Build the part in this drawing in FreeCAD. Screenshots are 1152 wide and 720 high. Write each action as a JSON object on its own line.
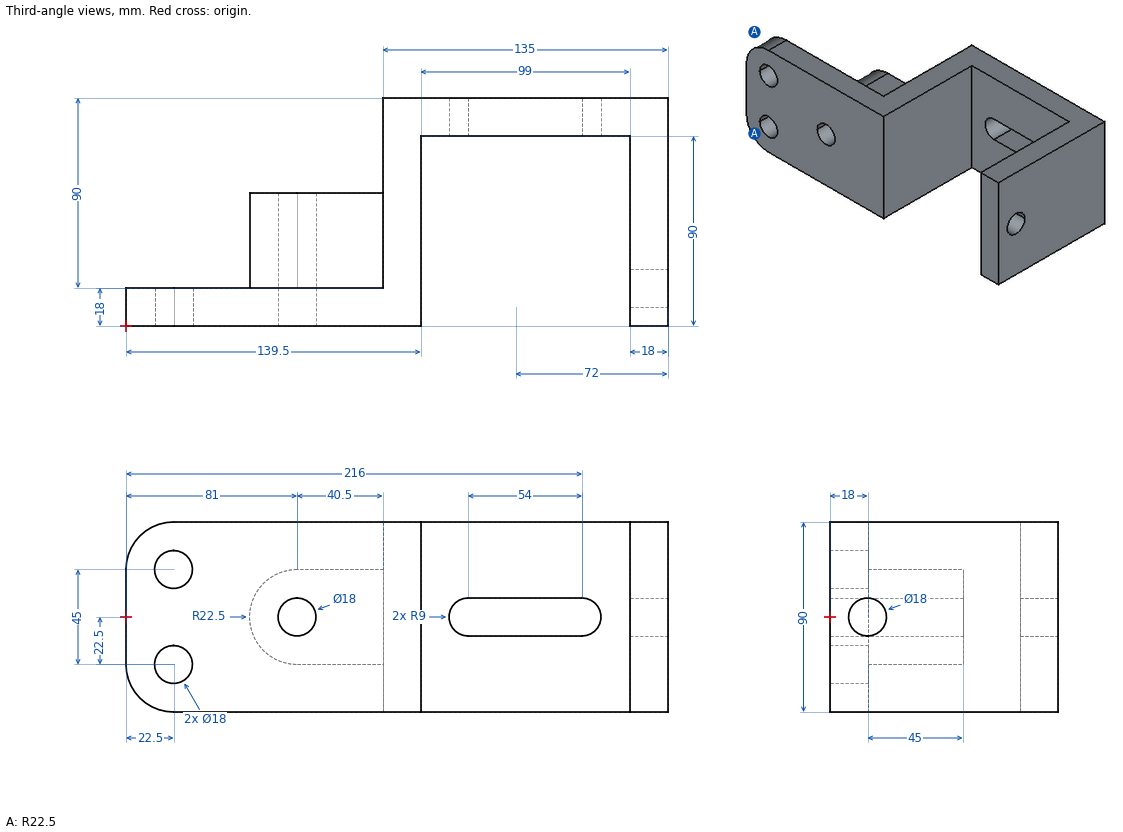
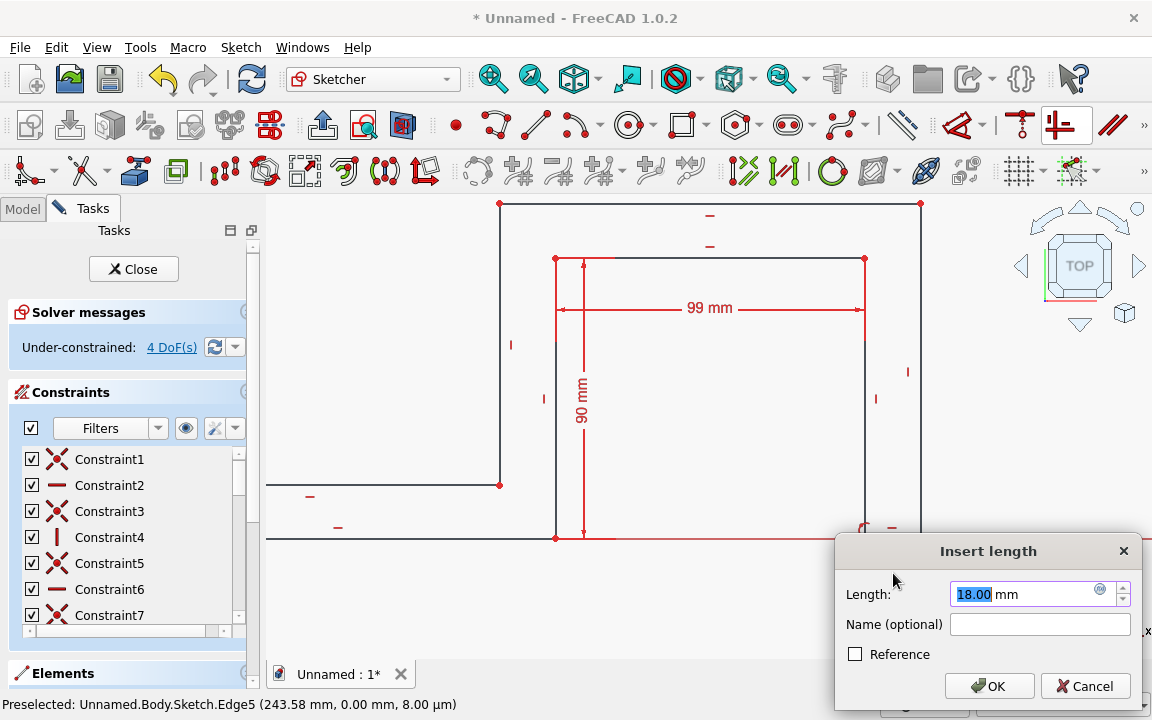
{"action": "type", "text": "18"}
{"action": "key", "text": "Return"}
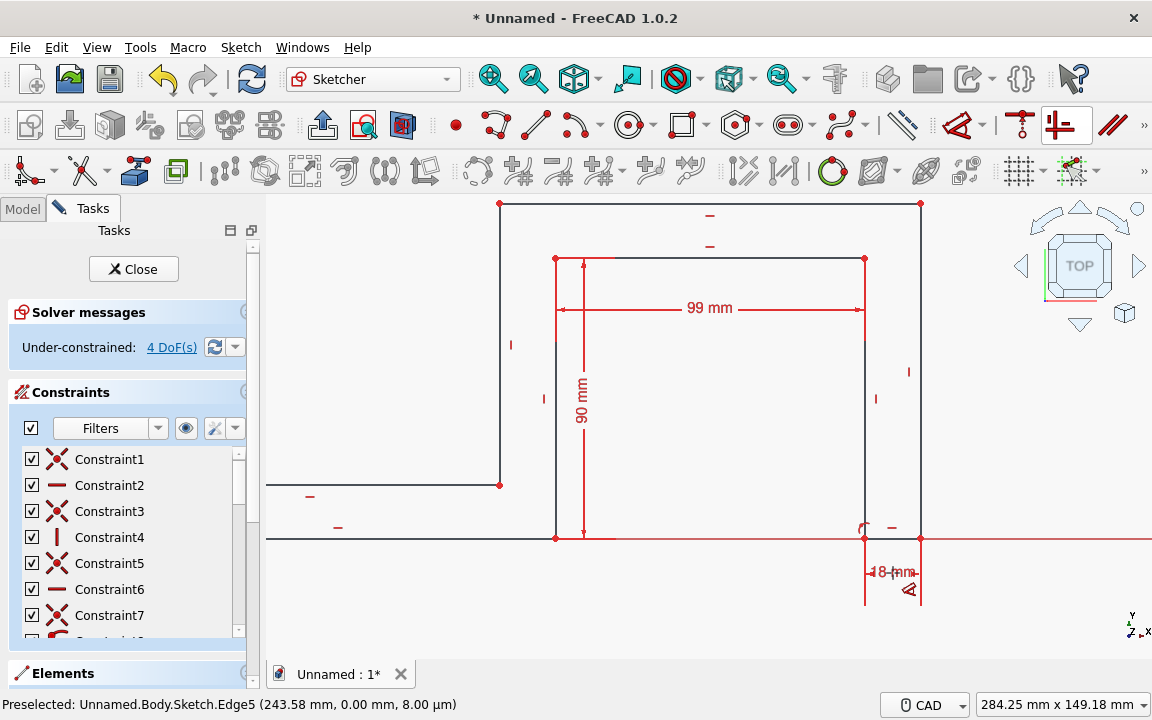
{"action": "left_click", "coordinate": [500, 288]}
{"action": "left_click", "coordinate": [466, 354]}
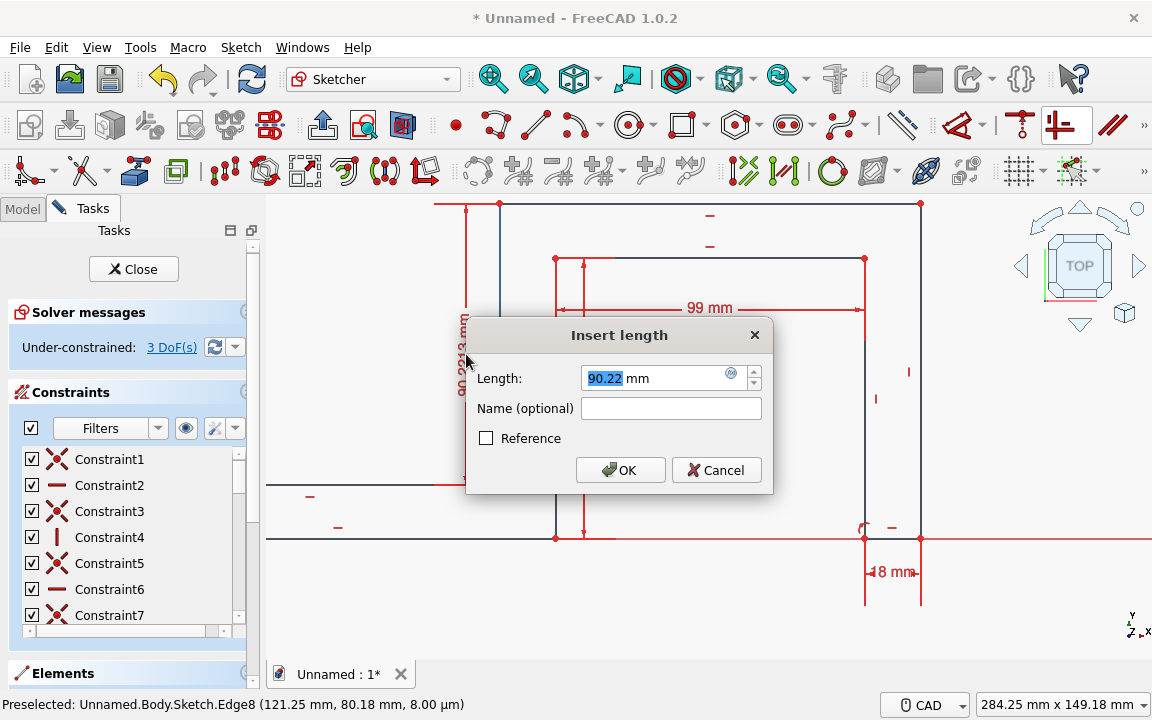
{"action": "type", "text": "90"}
{"action": "key", "text": "Return"}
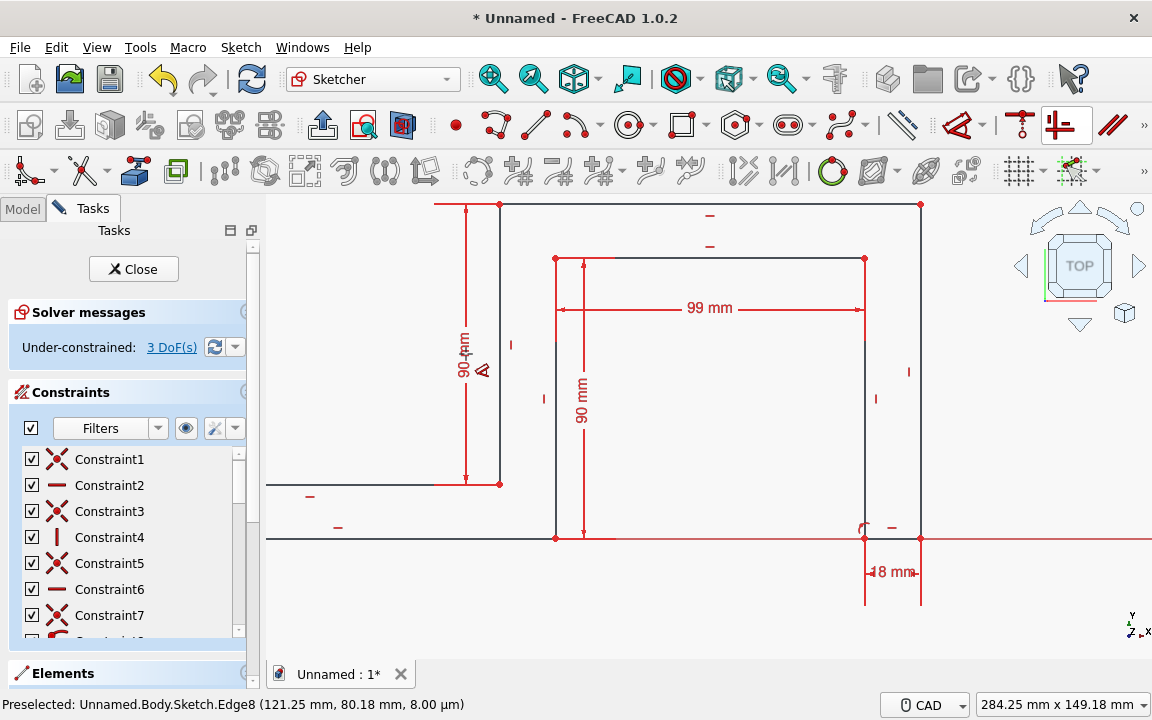
{"action": "scroll", "coordinate": [882, 540], "scroll_direction": "down", "scroll_amount": 2}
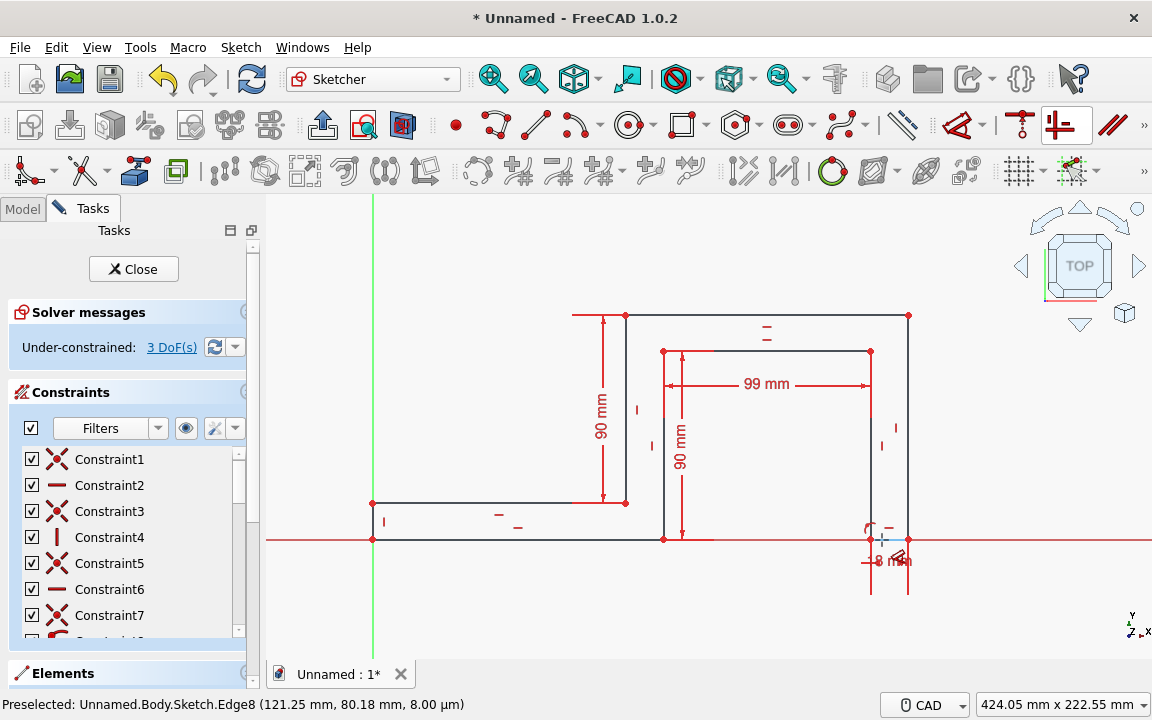
{"action": "scroll", "coordinate": [373, 514], "scroll_direction": "up", "scroll_amount": 2}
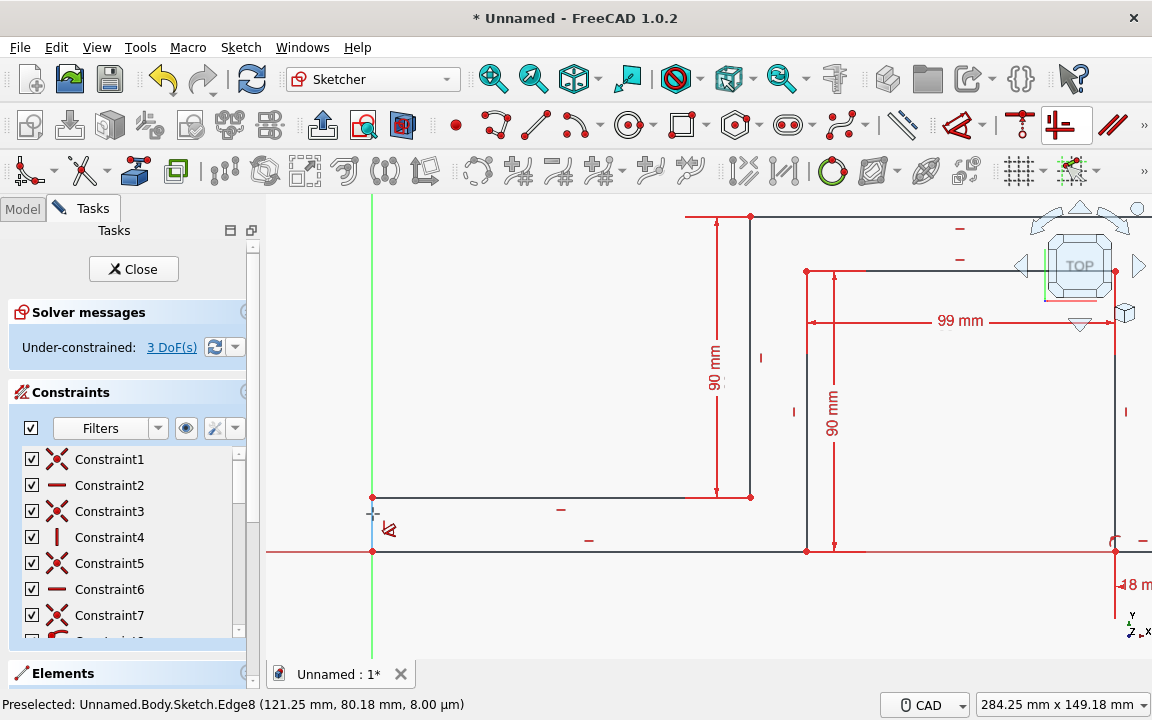
{"action": "left_click", "coordinate": [372, 514]}
{"action": "left_click", "coordinate": [338, 525]}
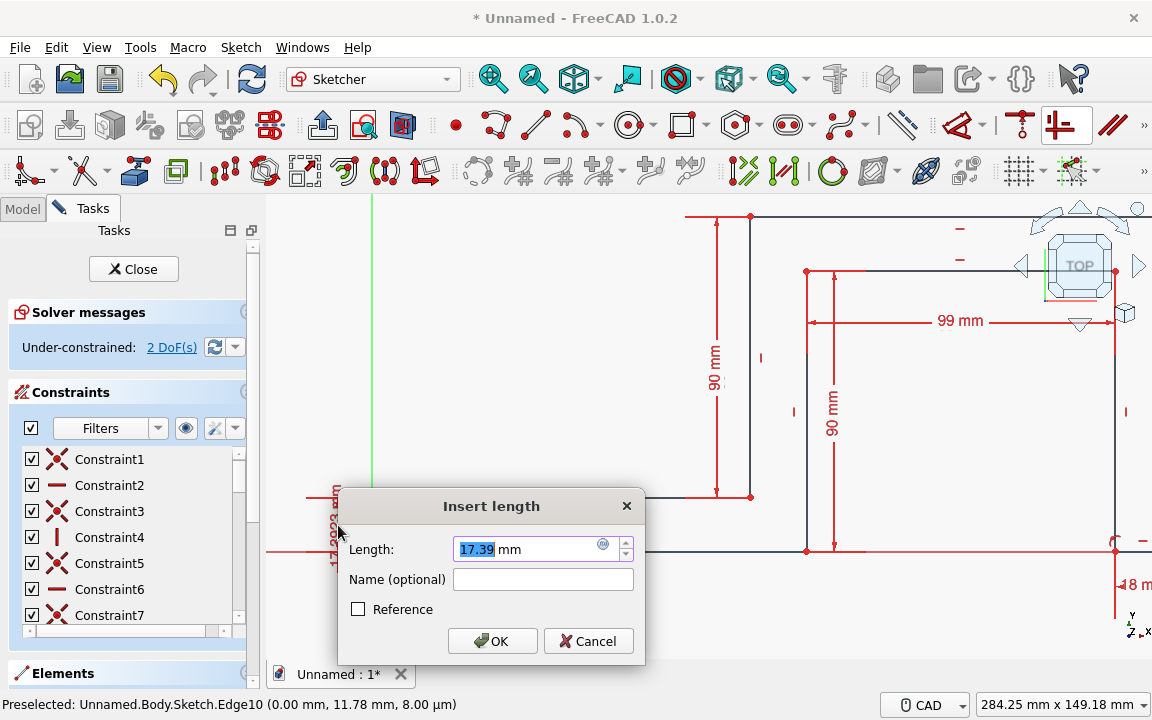
{"action": "type", "text": "18"}
{"action": "key", "text": "Return"}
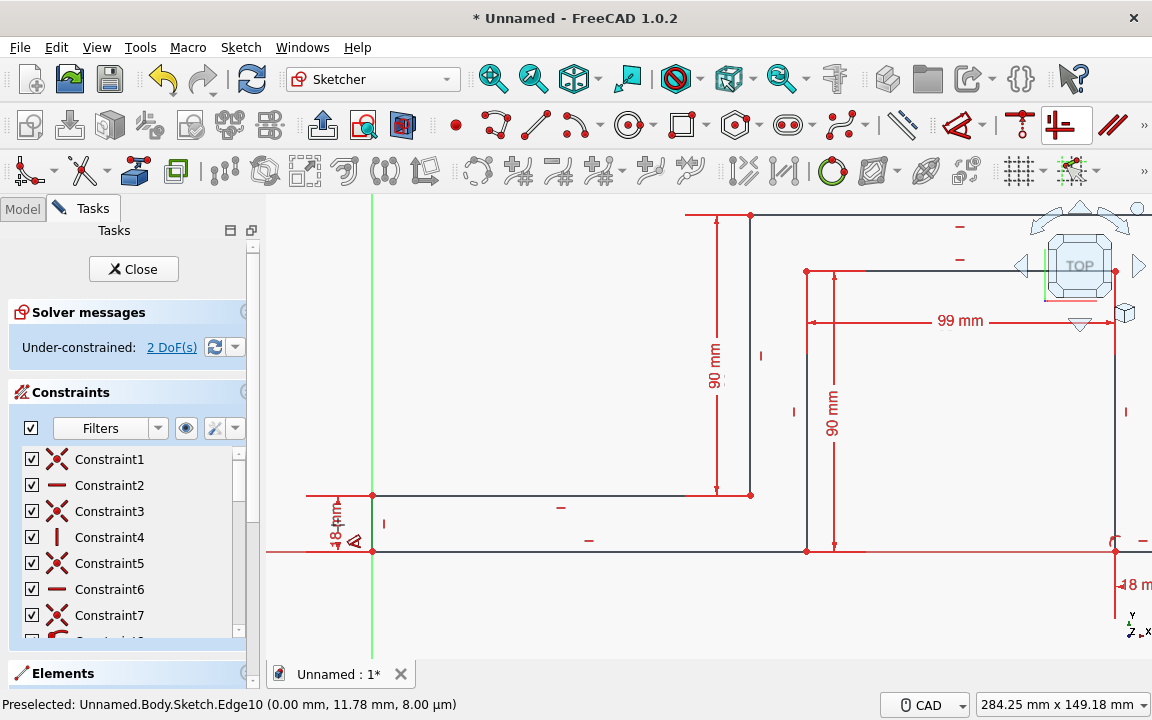
{"action": "scroll", "coordinate": [373, 514], "scroll_direction": "down", "scroll_amount": 2}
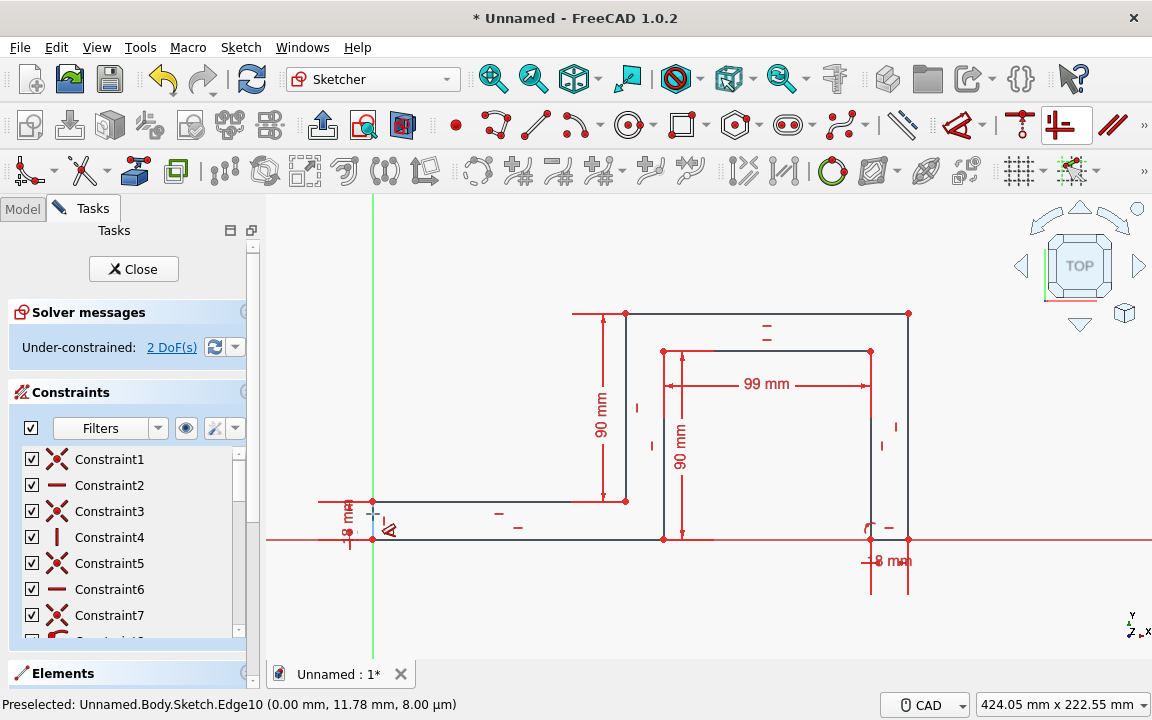
{"action": "left_click", "coordinate": [823, 314]}
{"action": "left_click", "coordinate": [767, 280]}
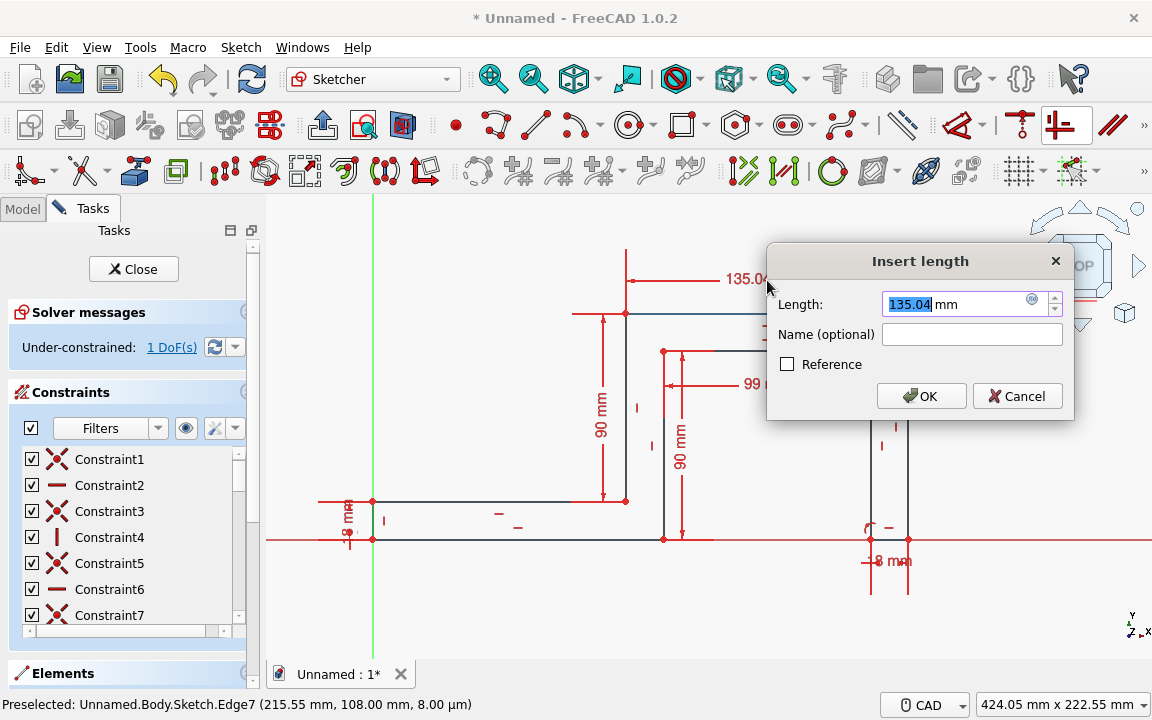
{"action": "type", "text": "135"}
{"action": "key", "text": "Return"}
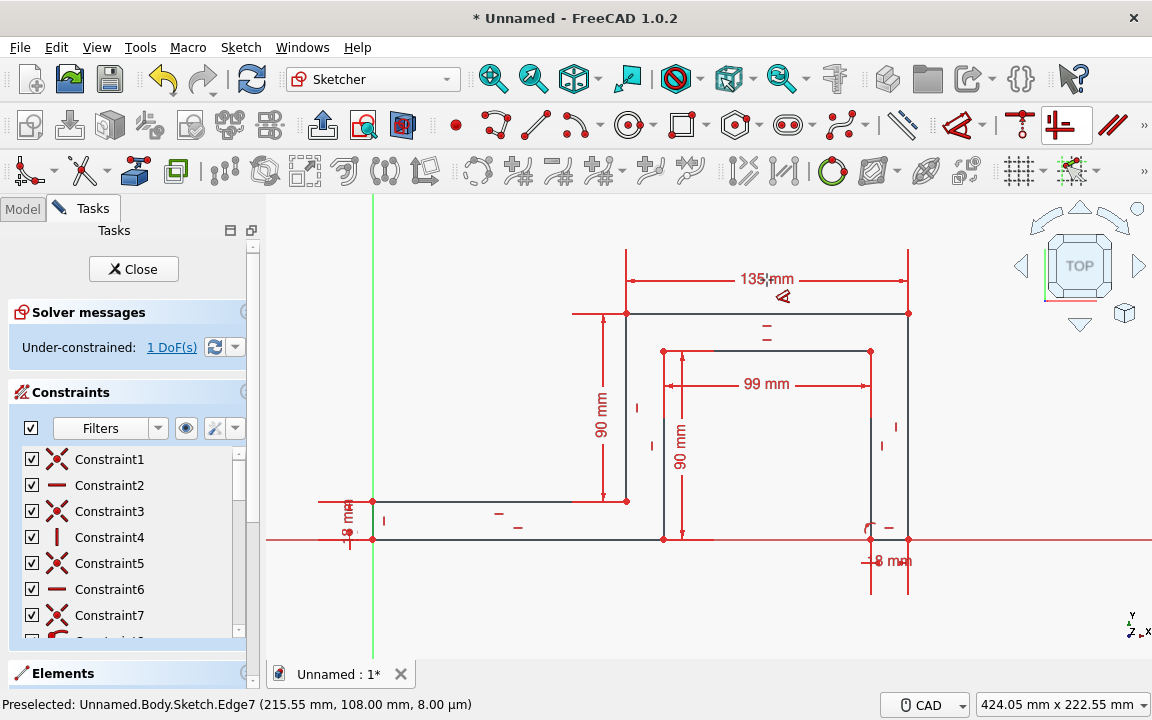
{"action": "left_click", "coordinate": [460, 540]}
{"action": "left_click", "coordinate": [518, 574]}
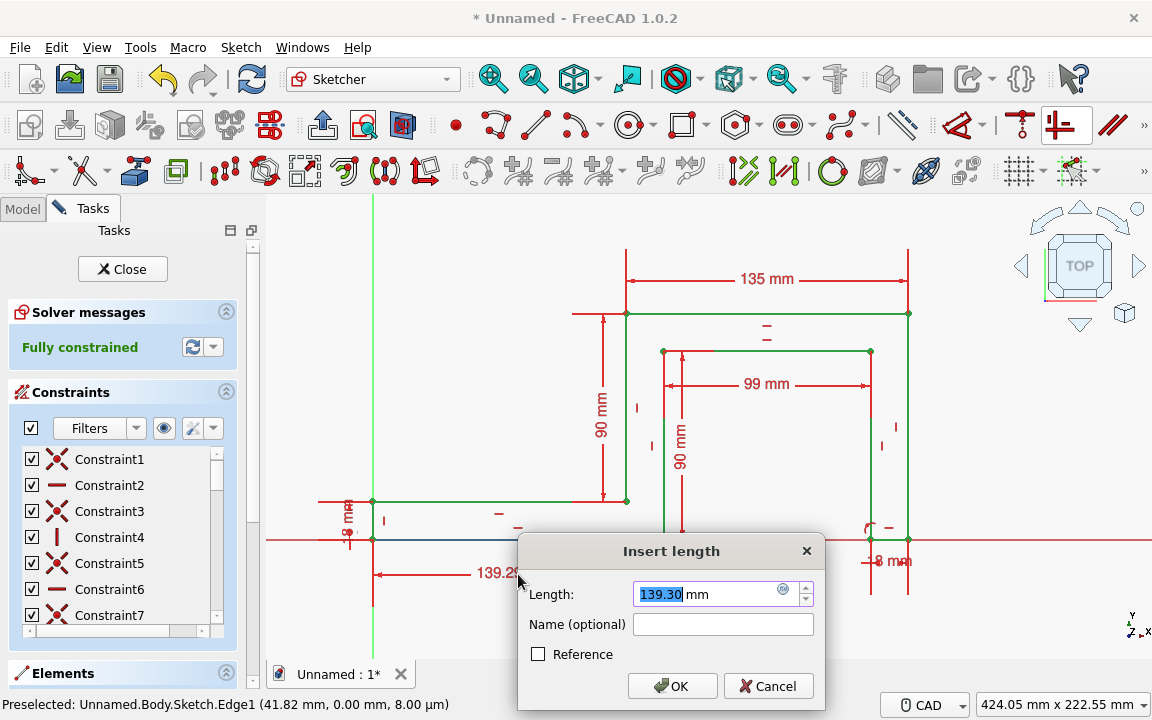
{"action": "type", "text": "139.5"}
{"action": "key", "text": "Return"}
{"action": "key", "text": "Escape"}